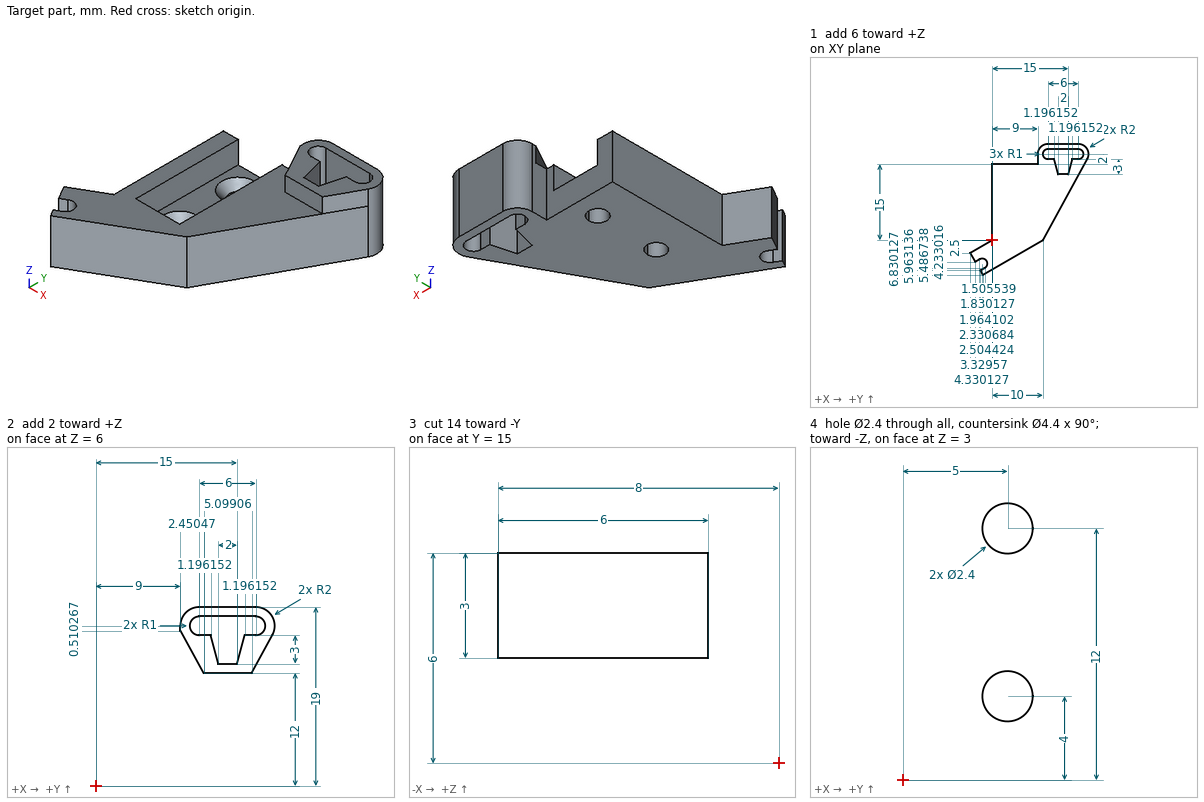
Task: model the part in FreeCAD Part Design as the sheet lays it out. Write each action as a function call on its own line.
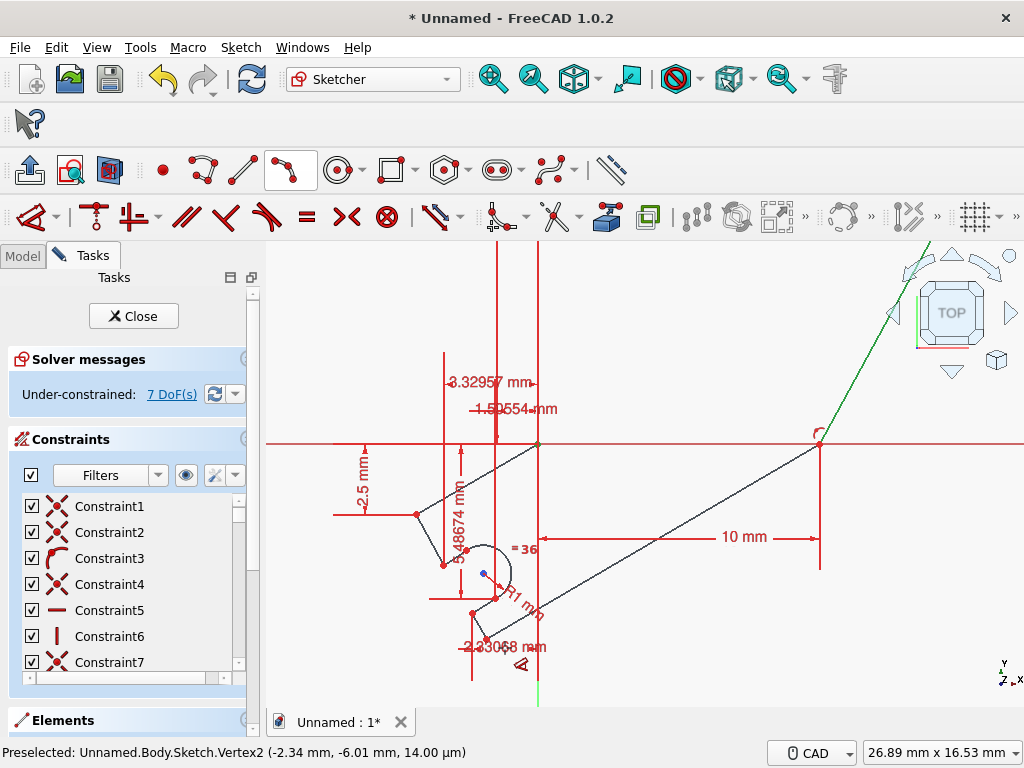
click(472, 614)
click(438, 470)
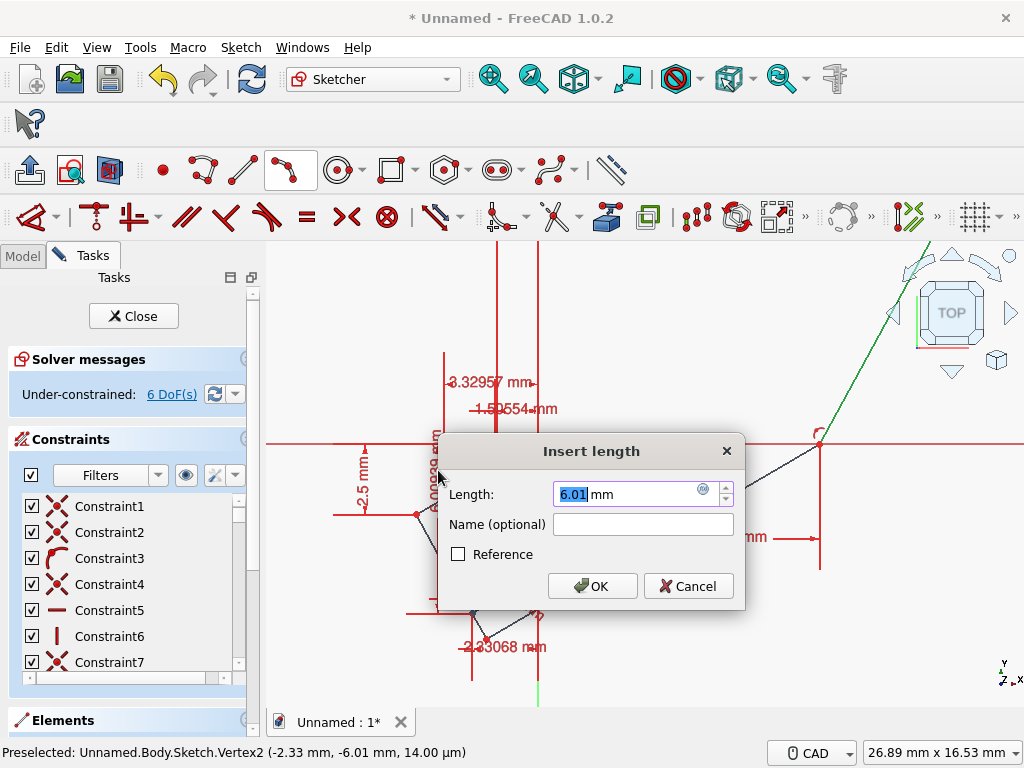
text(5.963136)
key(Return)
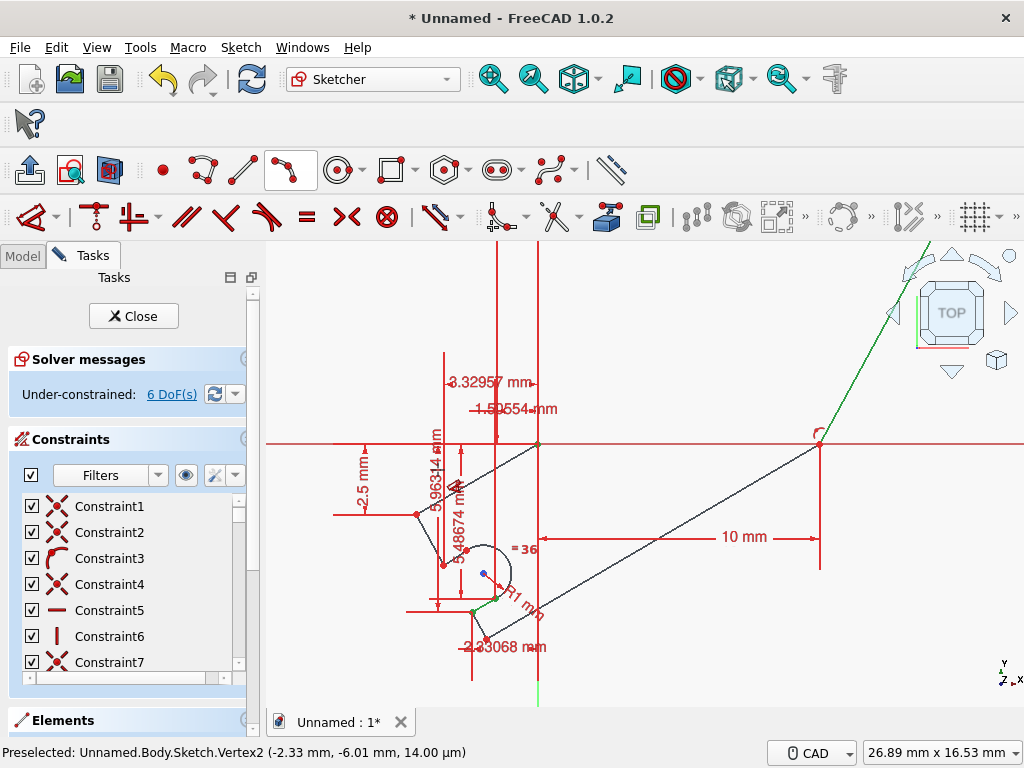
click(487, 639)
click(512, 673)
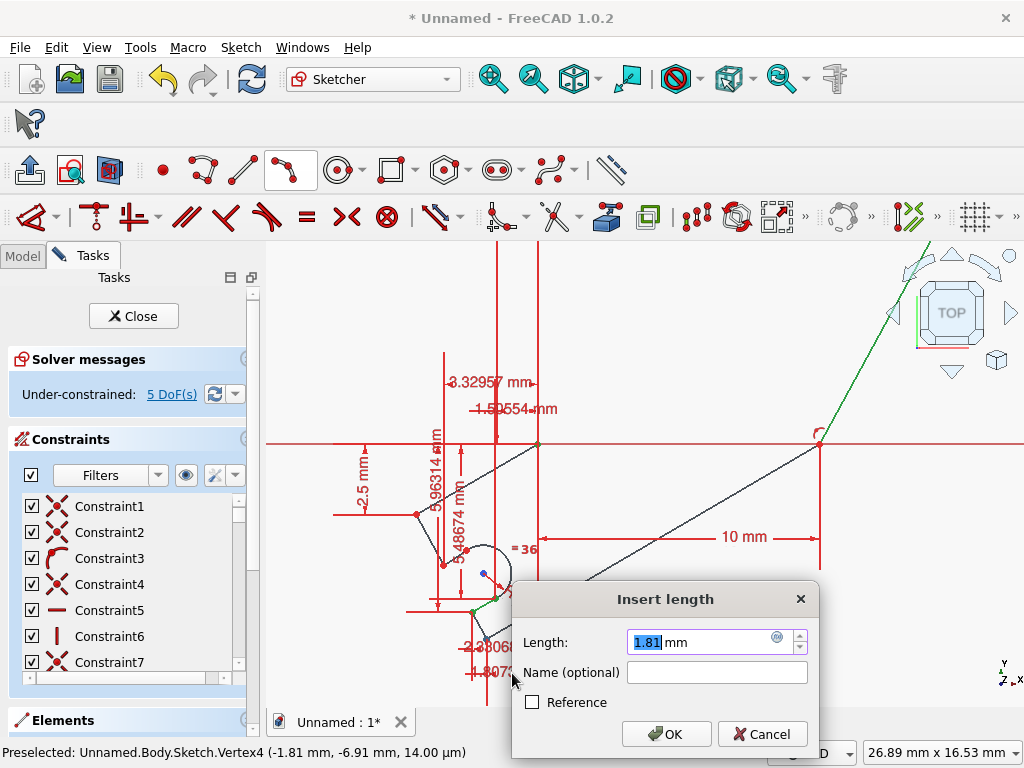
text(1.830127)
key(Return)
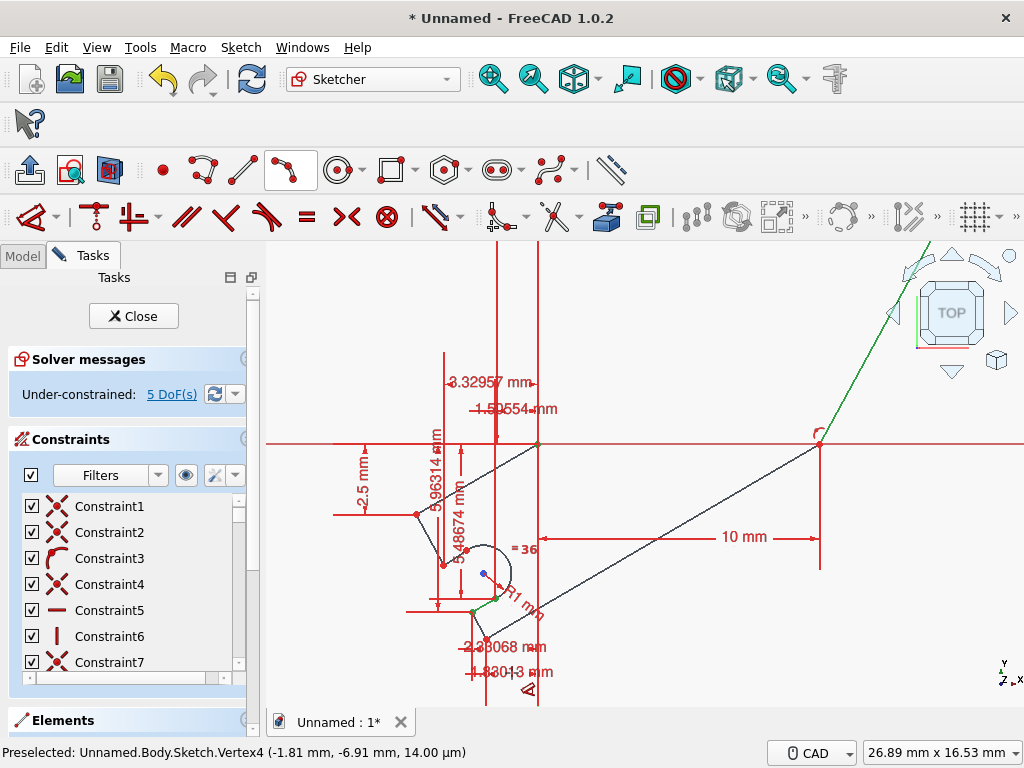
click(486, 639)
click(452, 586)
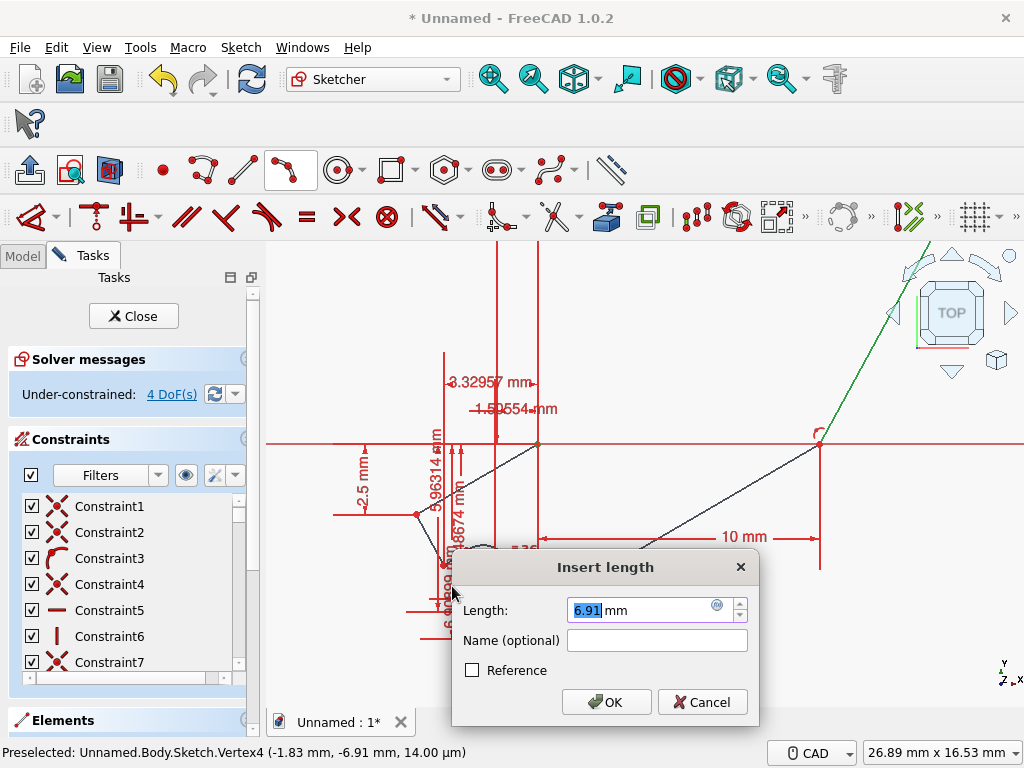
text(6.830127)
key(Return)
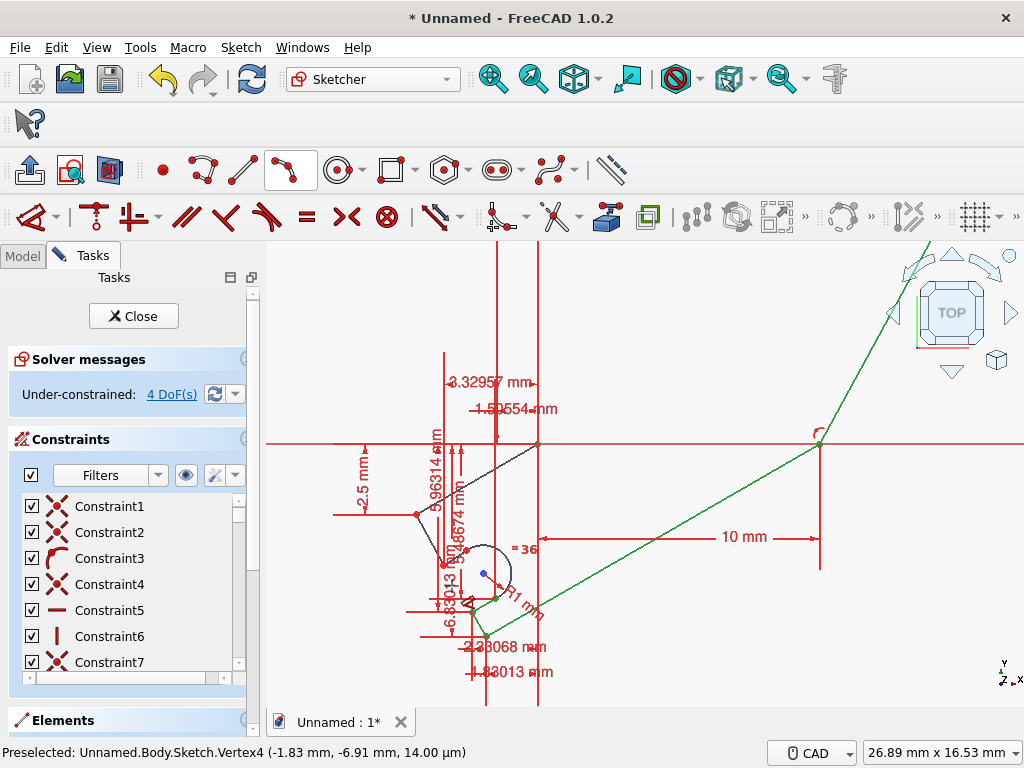
click(416, 515)
click(520, 549)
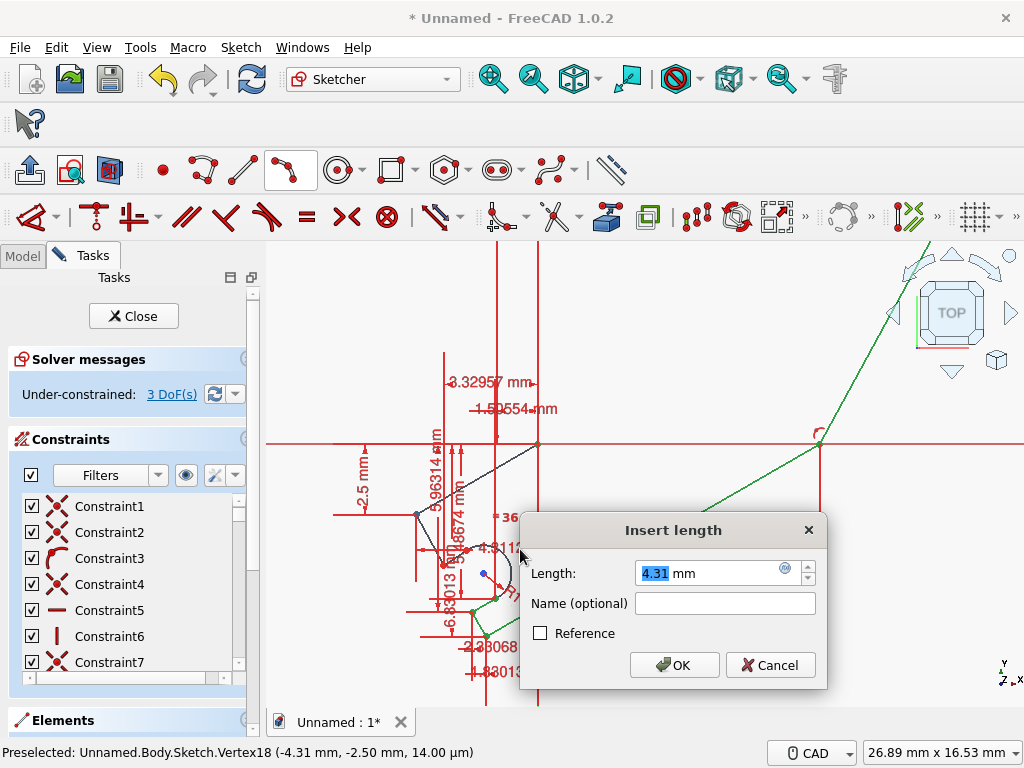
text(4.330127)
key(Return)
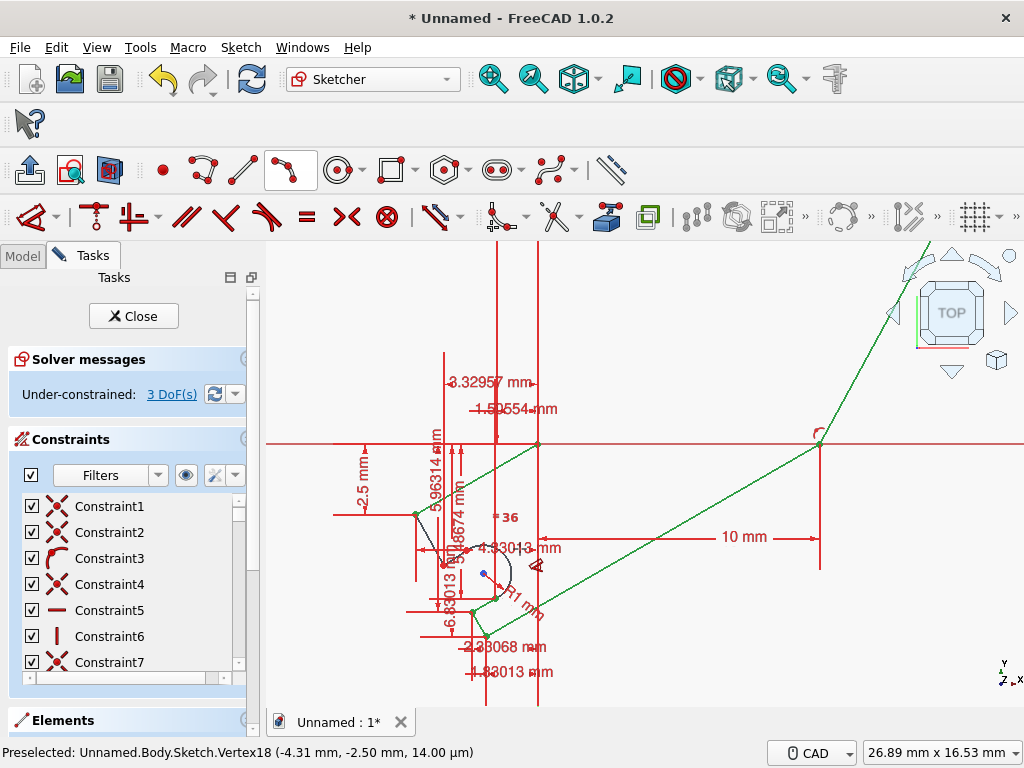
click(444, 566)
click(410, 547)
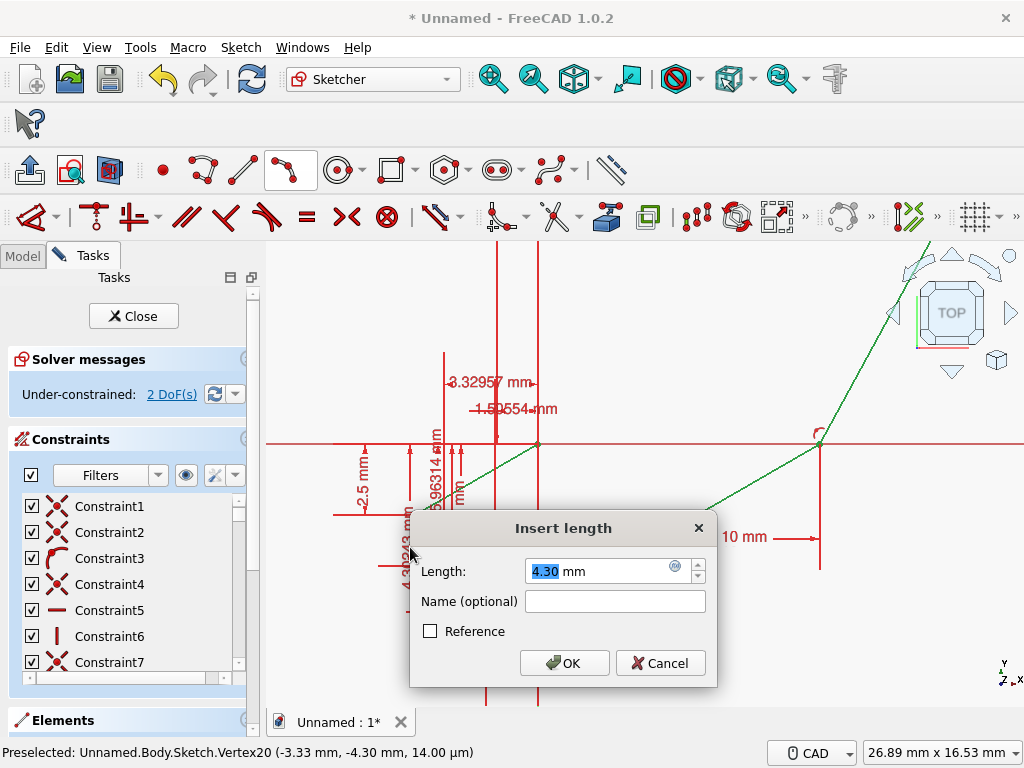
text(4.233016)
key(Return)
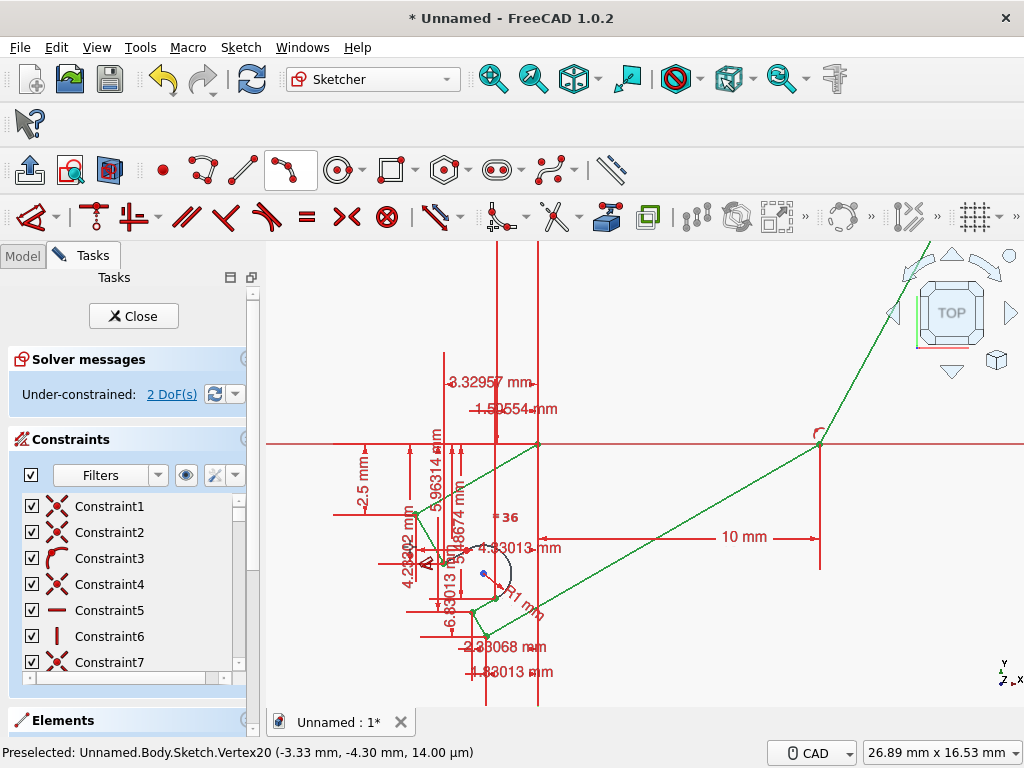
click(466, 551)
click(502, 362)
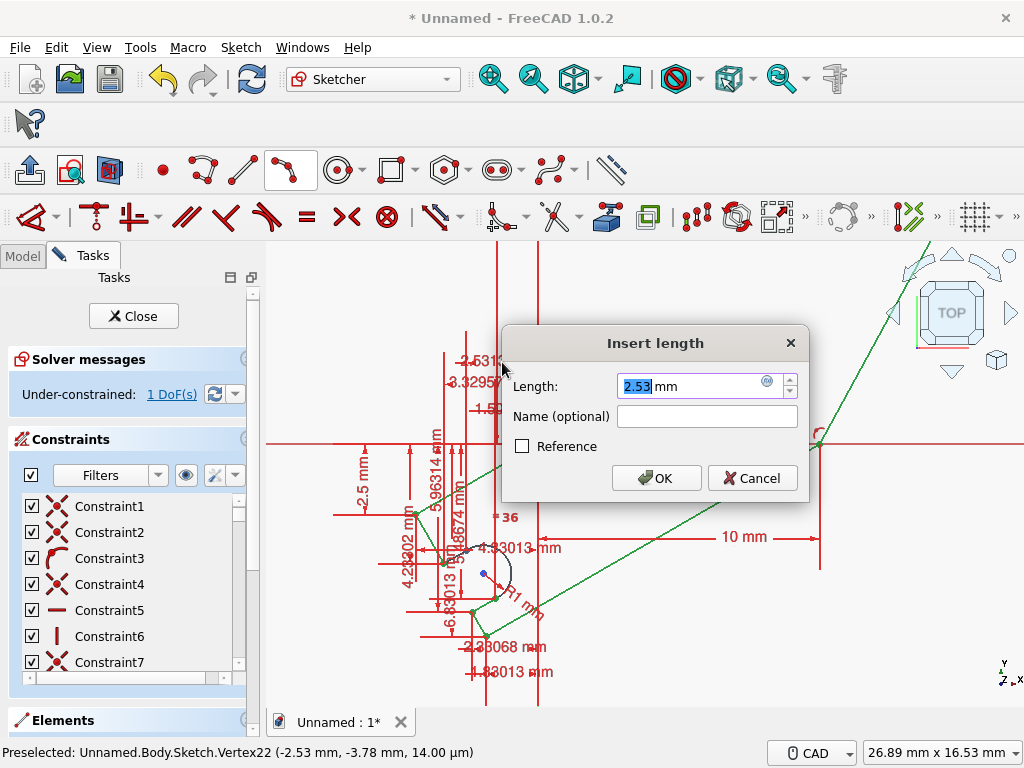
text(2.504424)
key(Return)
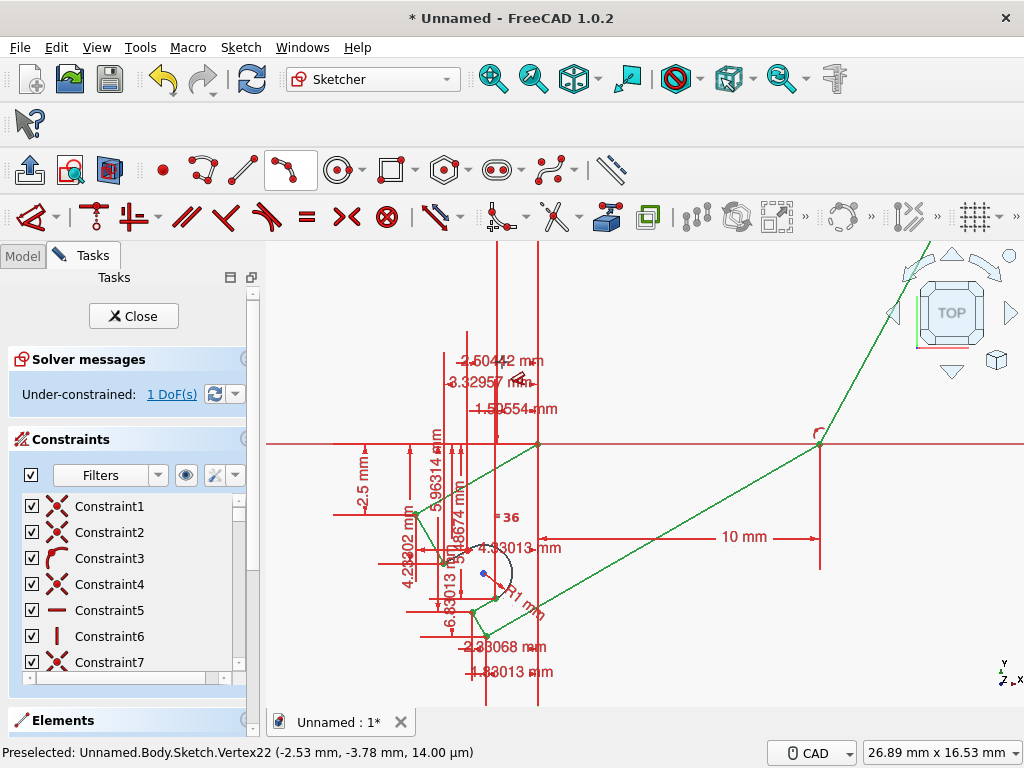
click(484, 573)
click(511, 338)